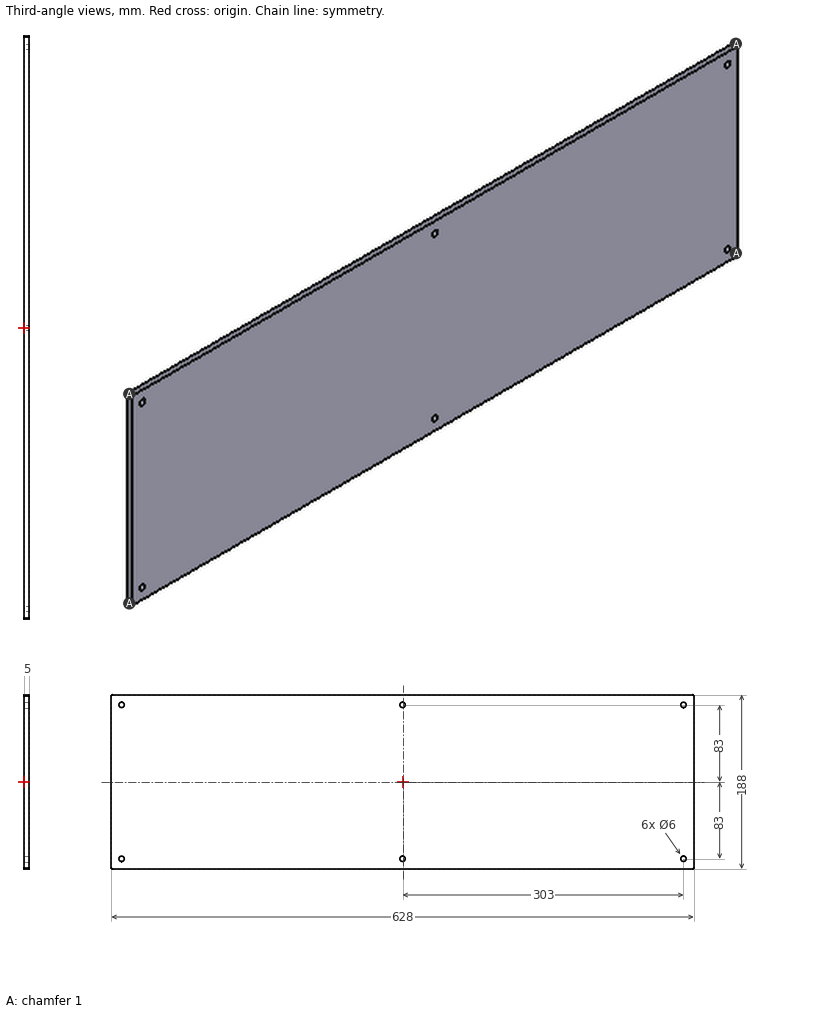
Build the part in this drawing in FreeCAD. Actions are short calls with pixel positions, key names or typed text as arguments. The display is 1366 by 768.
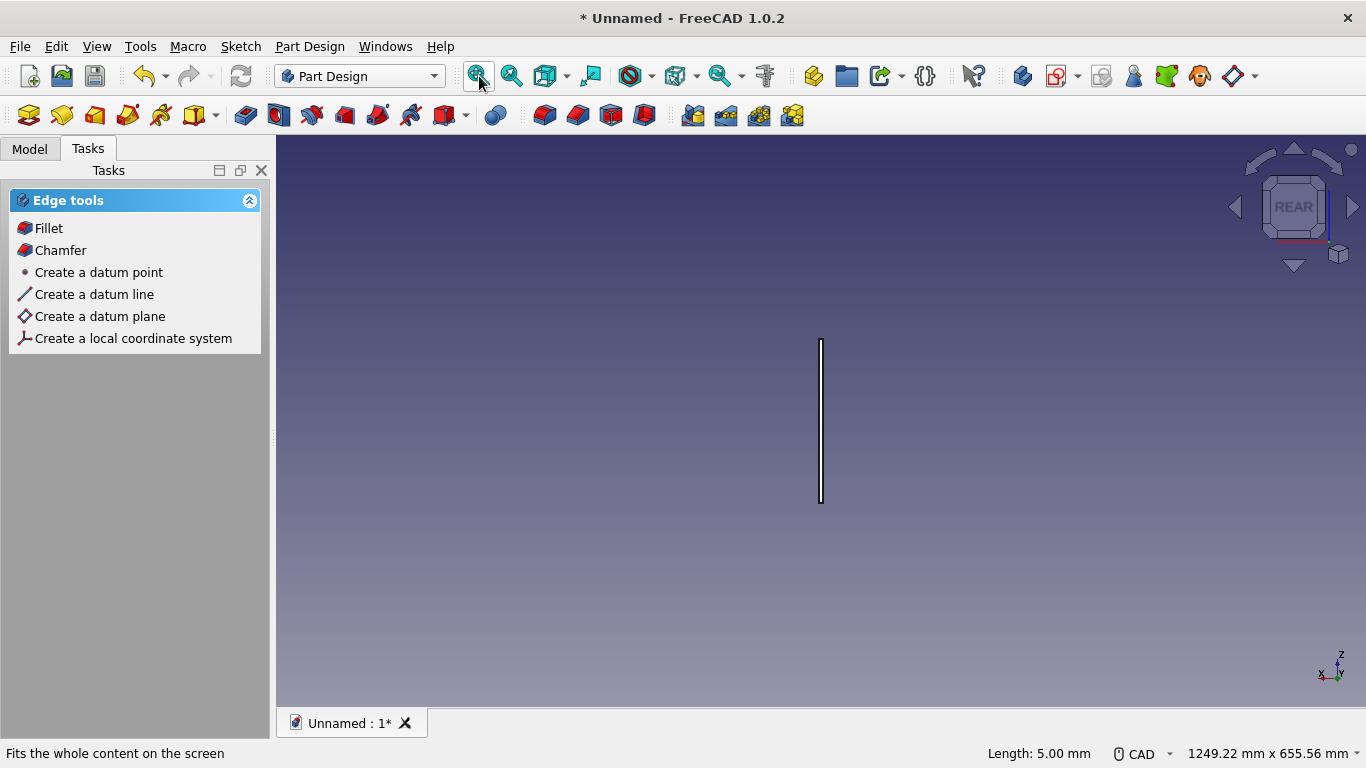
scroll(821, 338, up, 12)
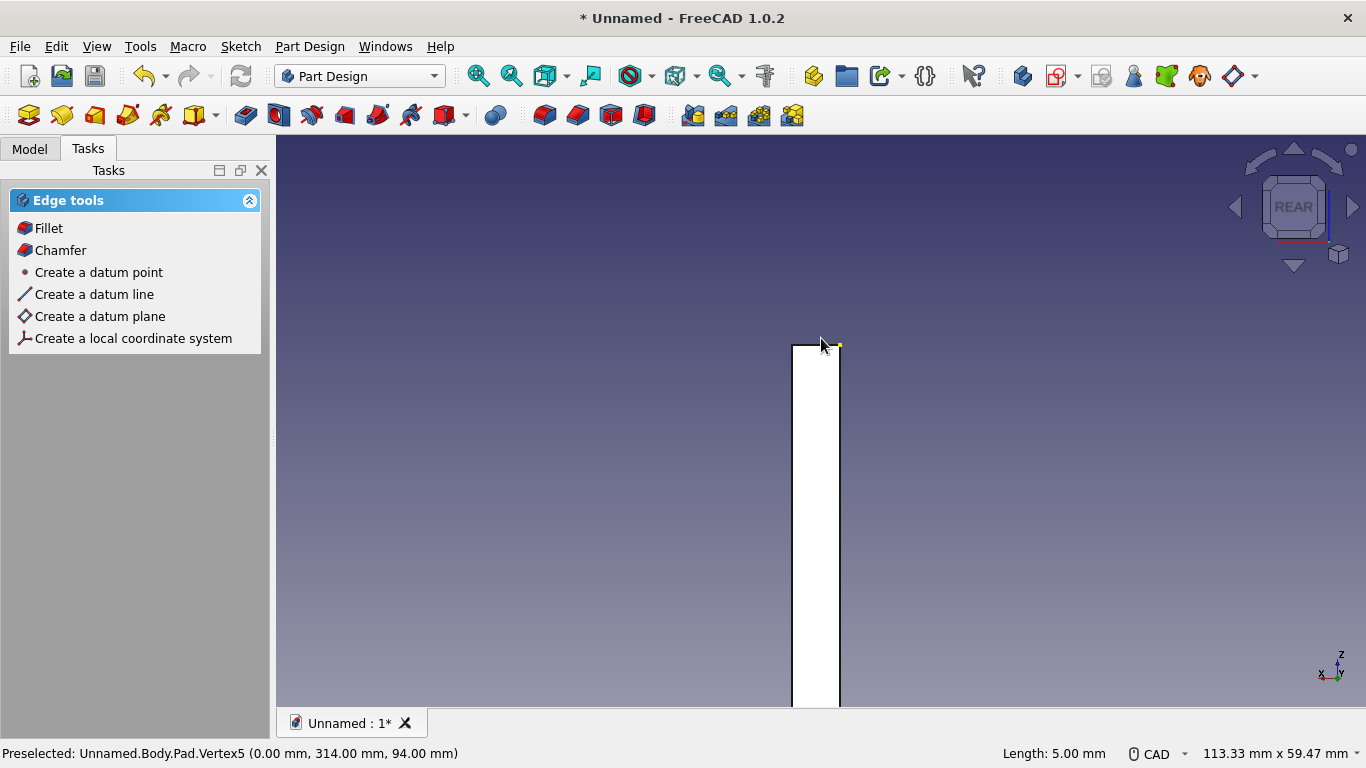
click(816, 344, ctrl)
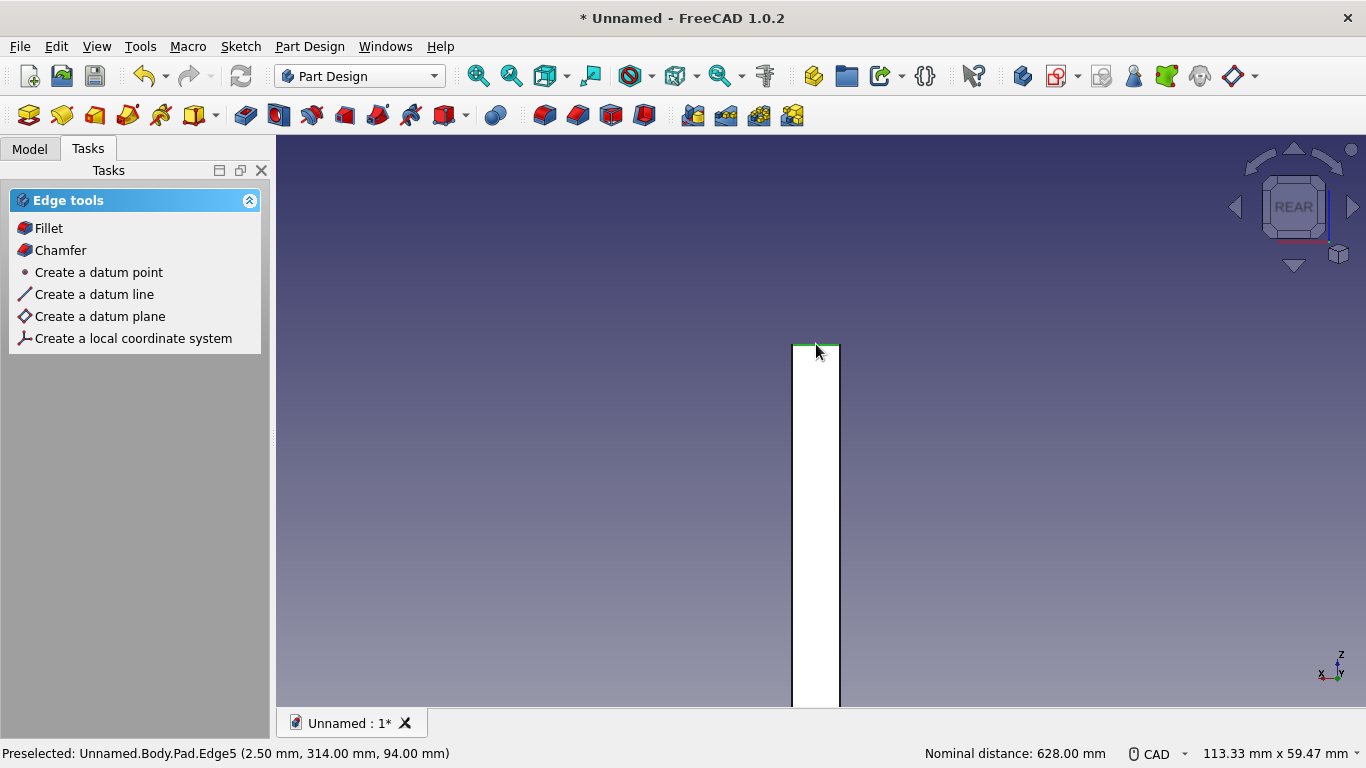
click(479, 76)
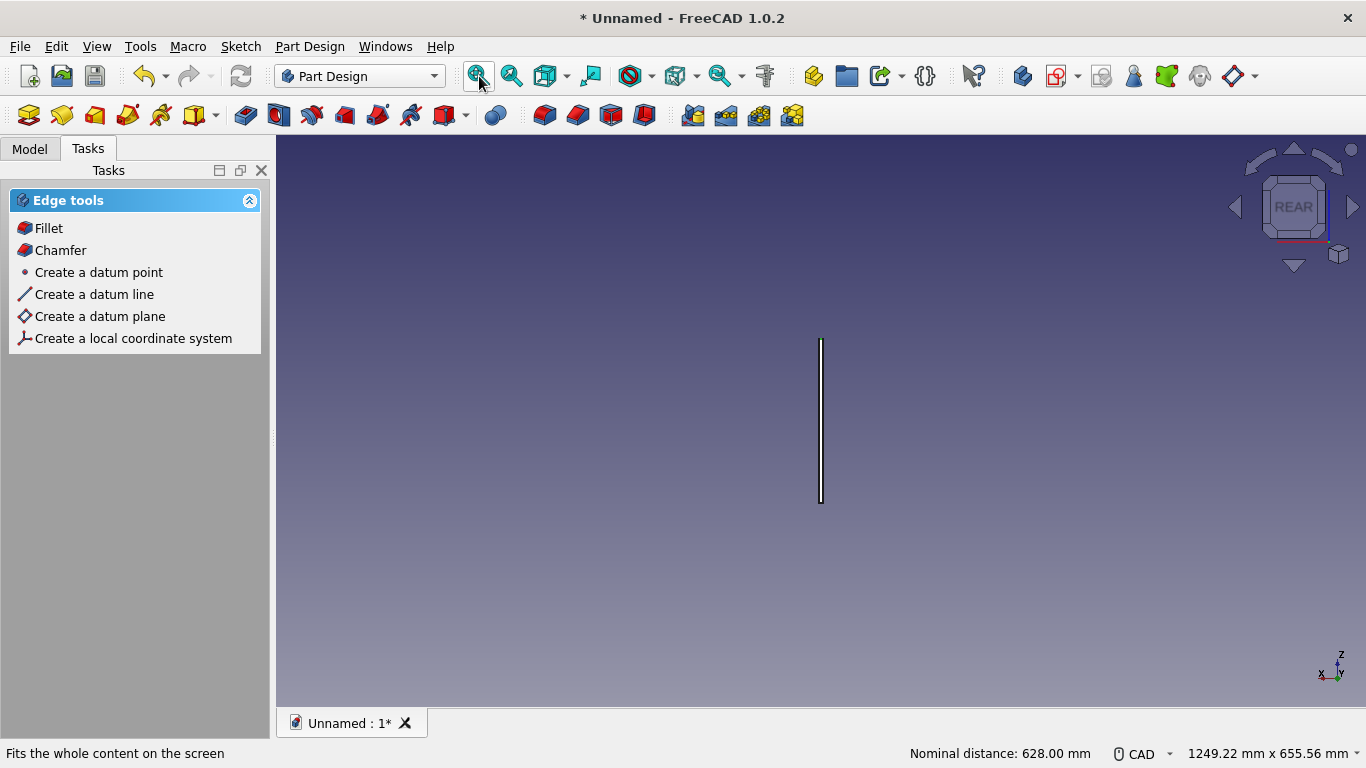
key(6)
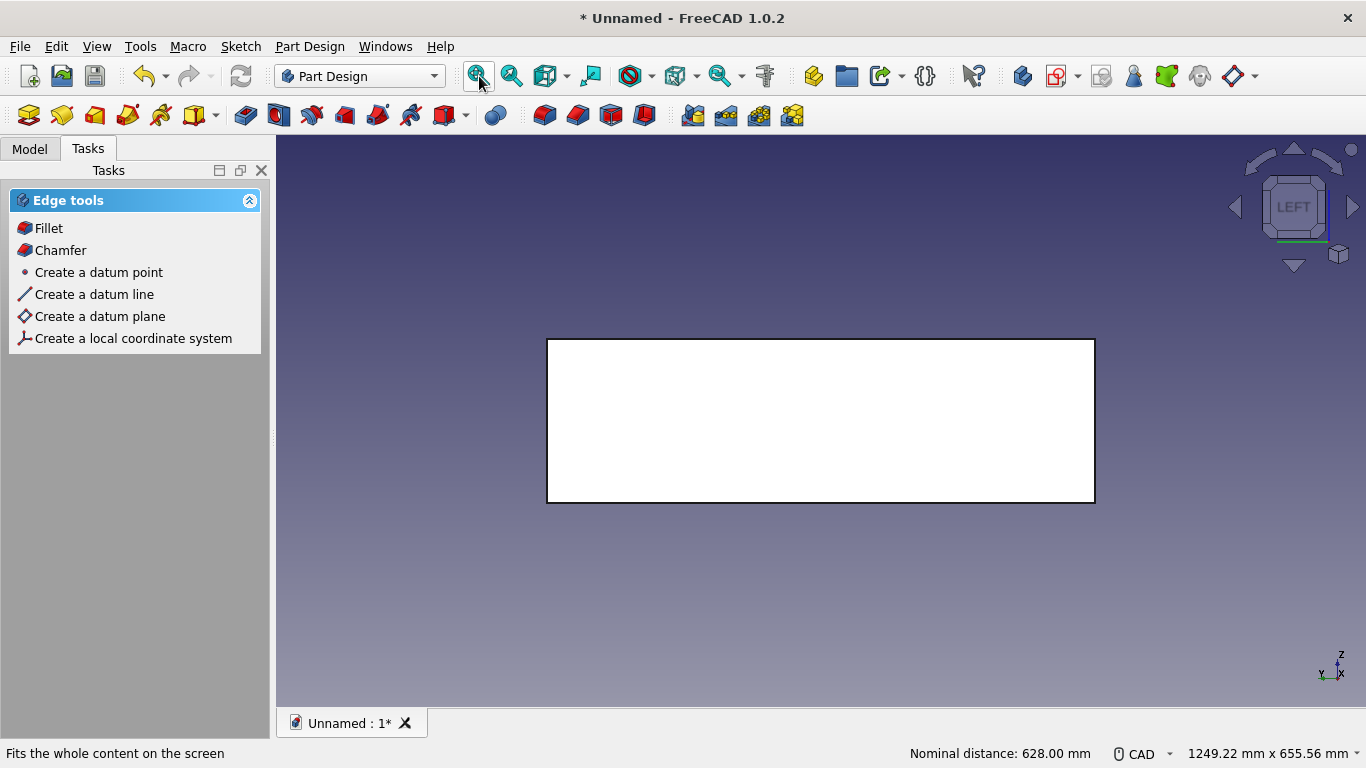
scroll(547, 502, up, 12)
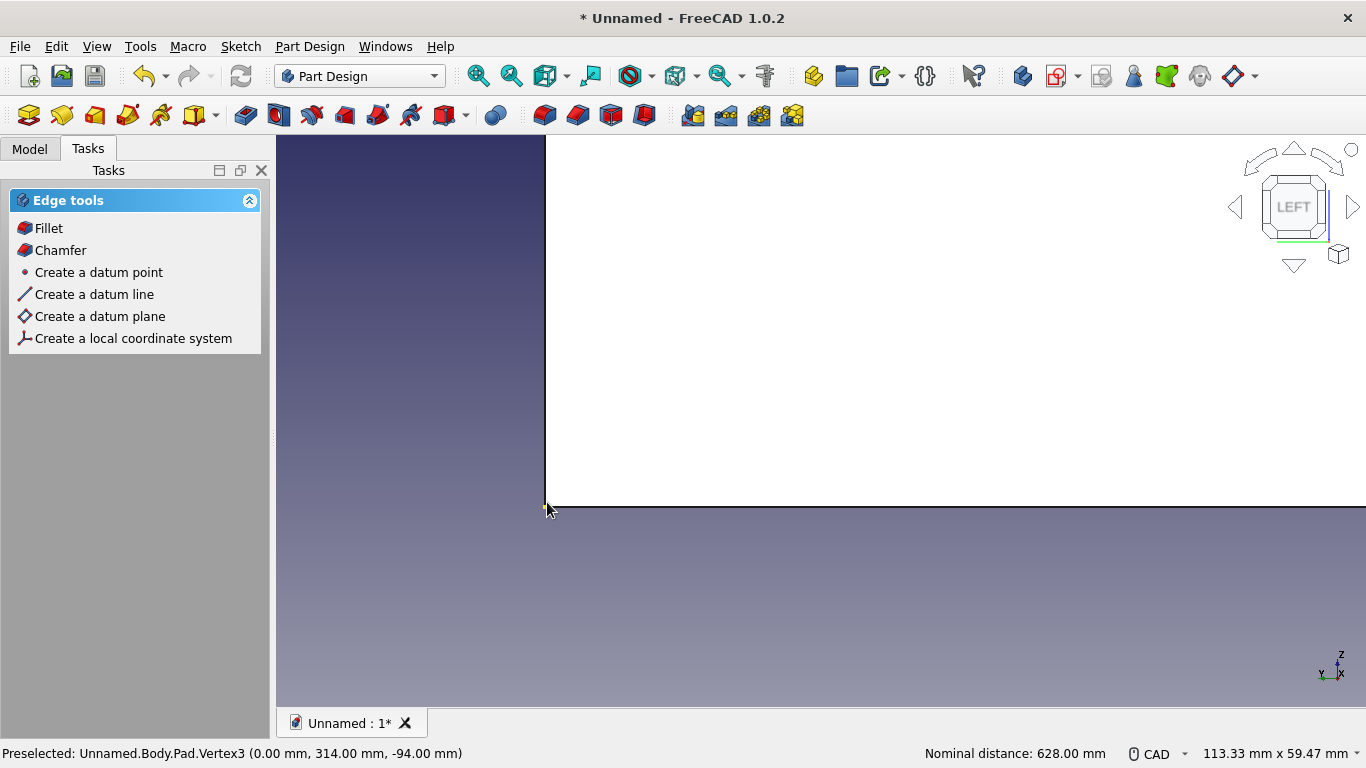
click(479, 76)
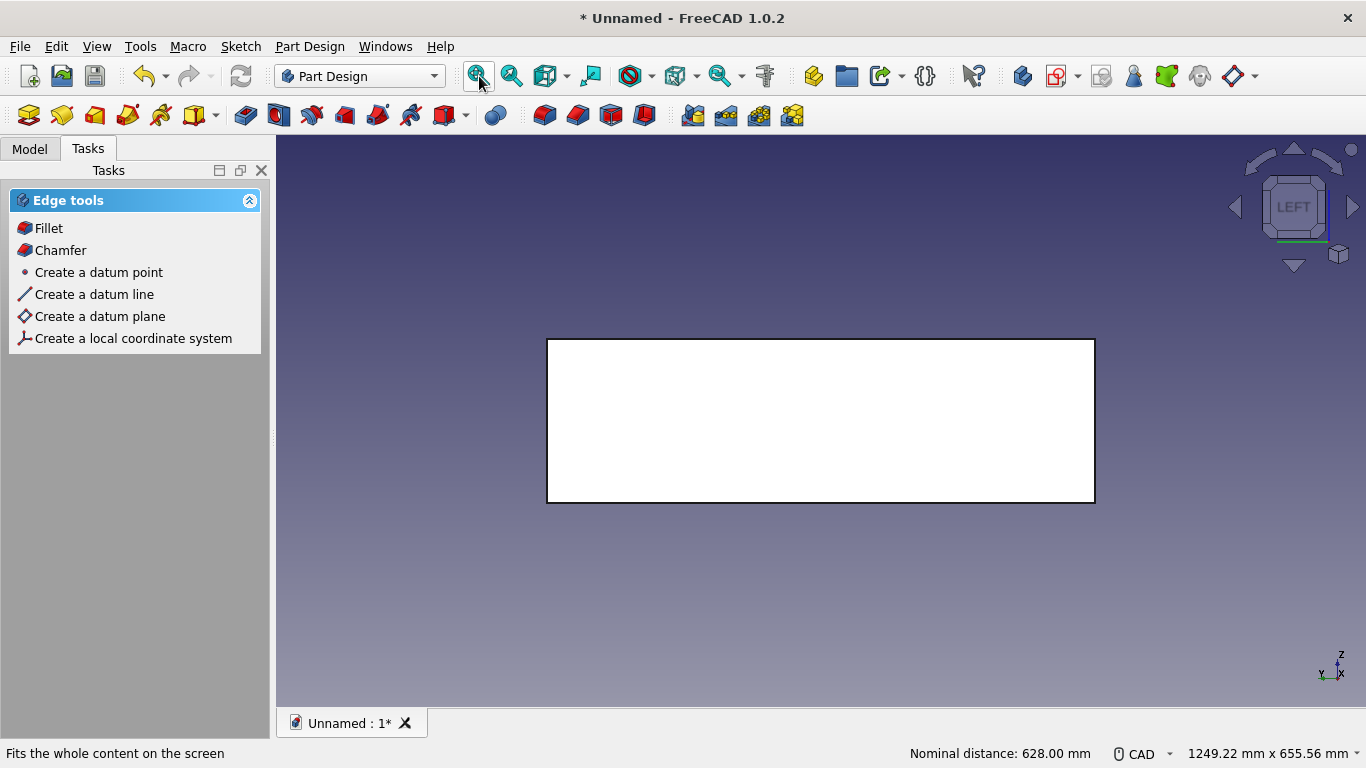
key(v)
key(3)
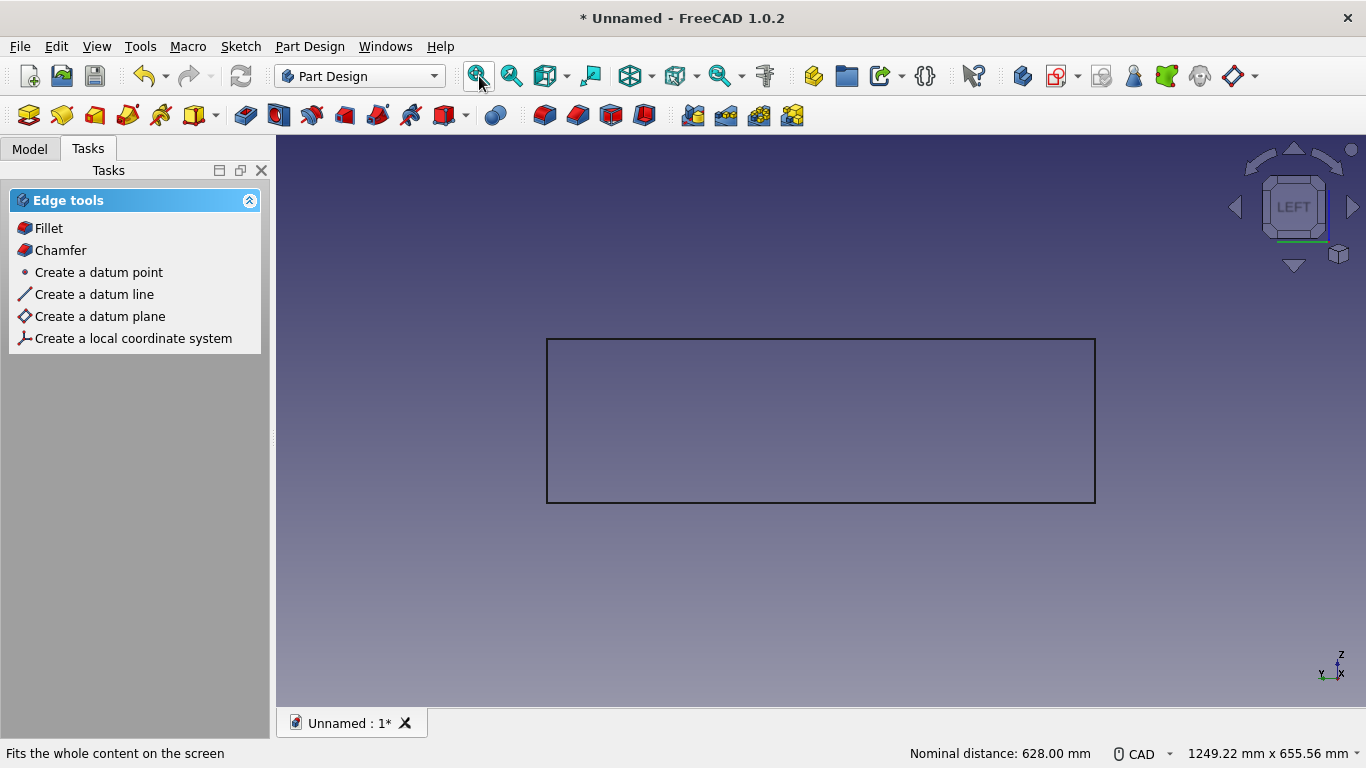
key(0)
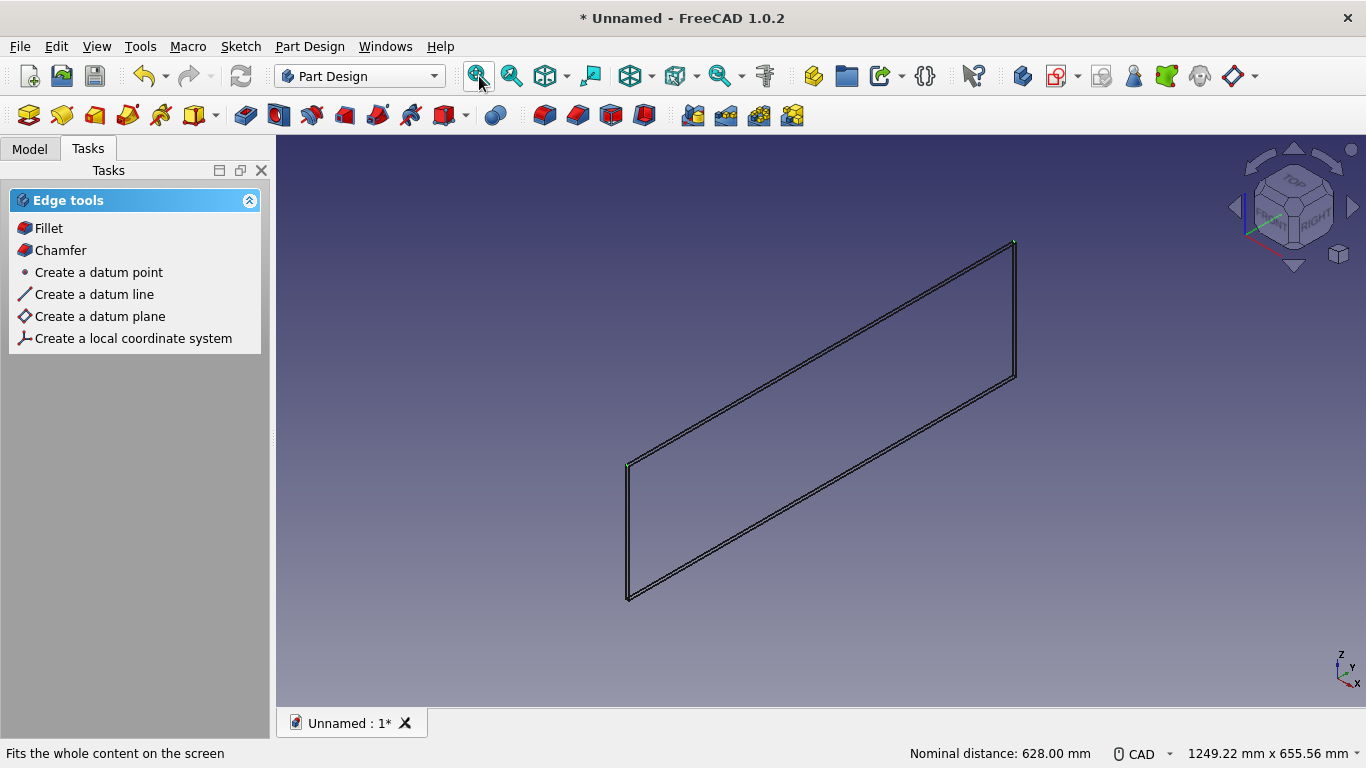
scroll(1015, 375, up, 12)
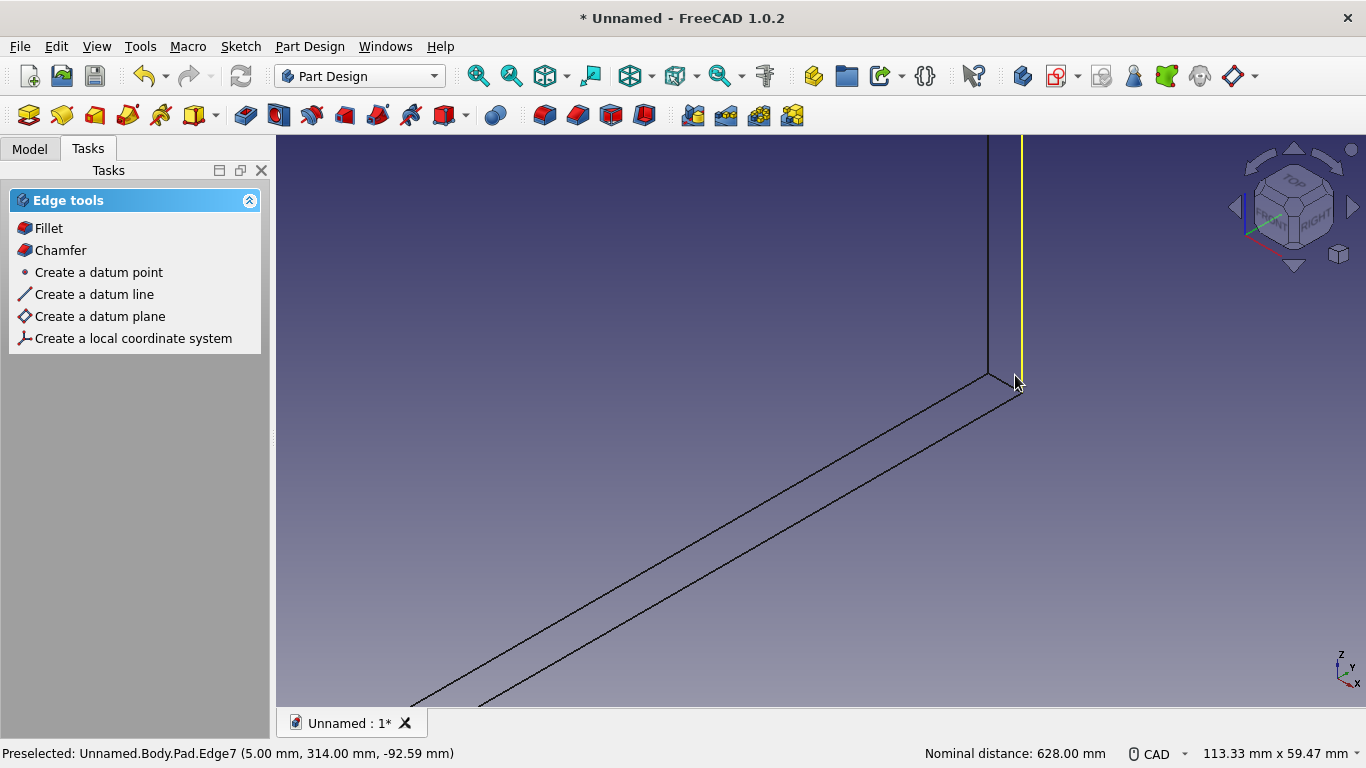
click(1005, 382, ctrl)